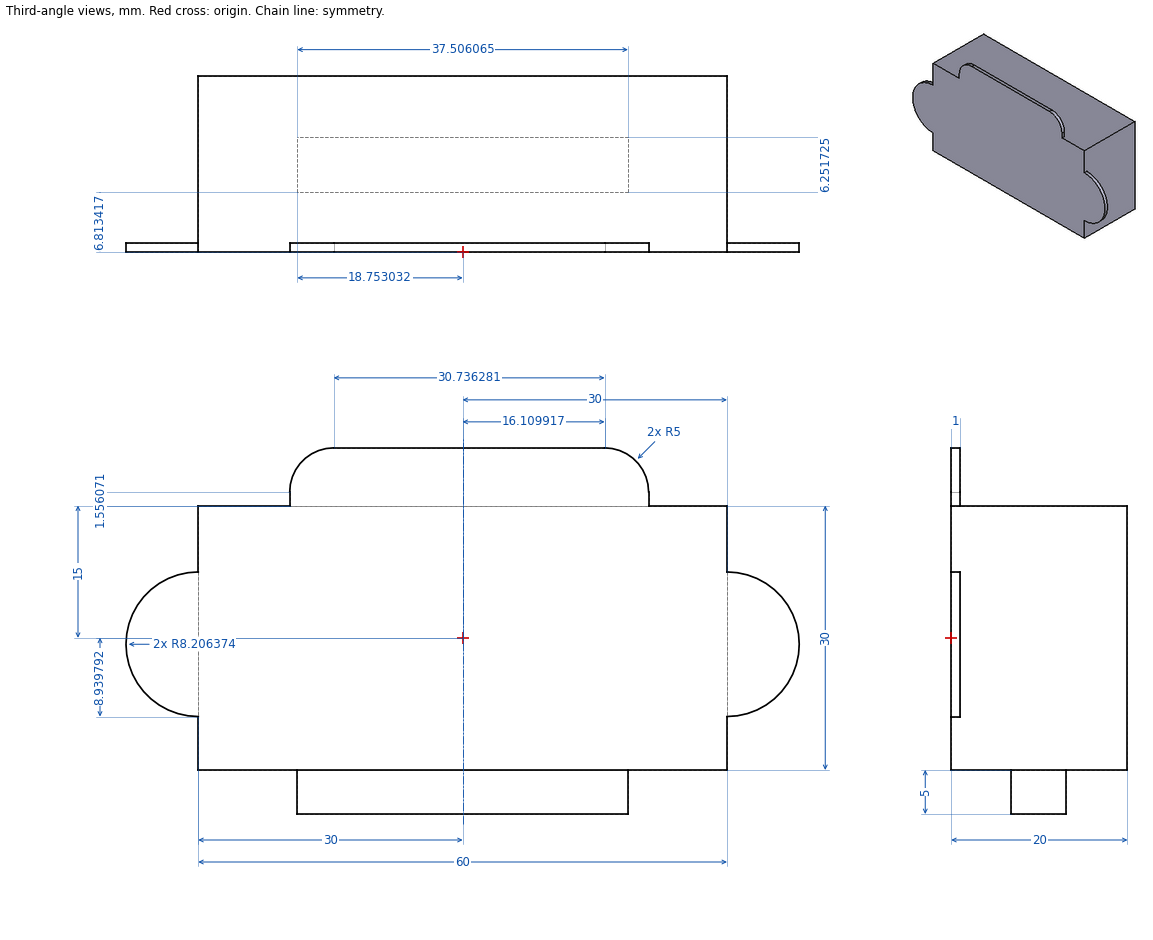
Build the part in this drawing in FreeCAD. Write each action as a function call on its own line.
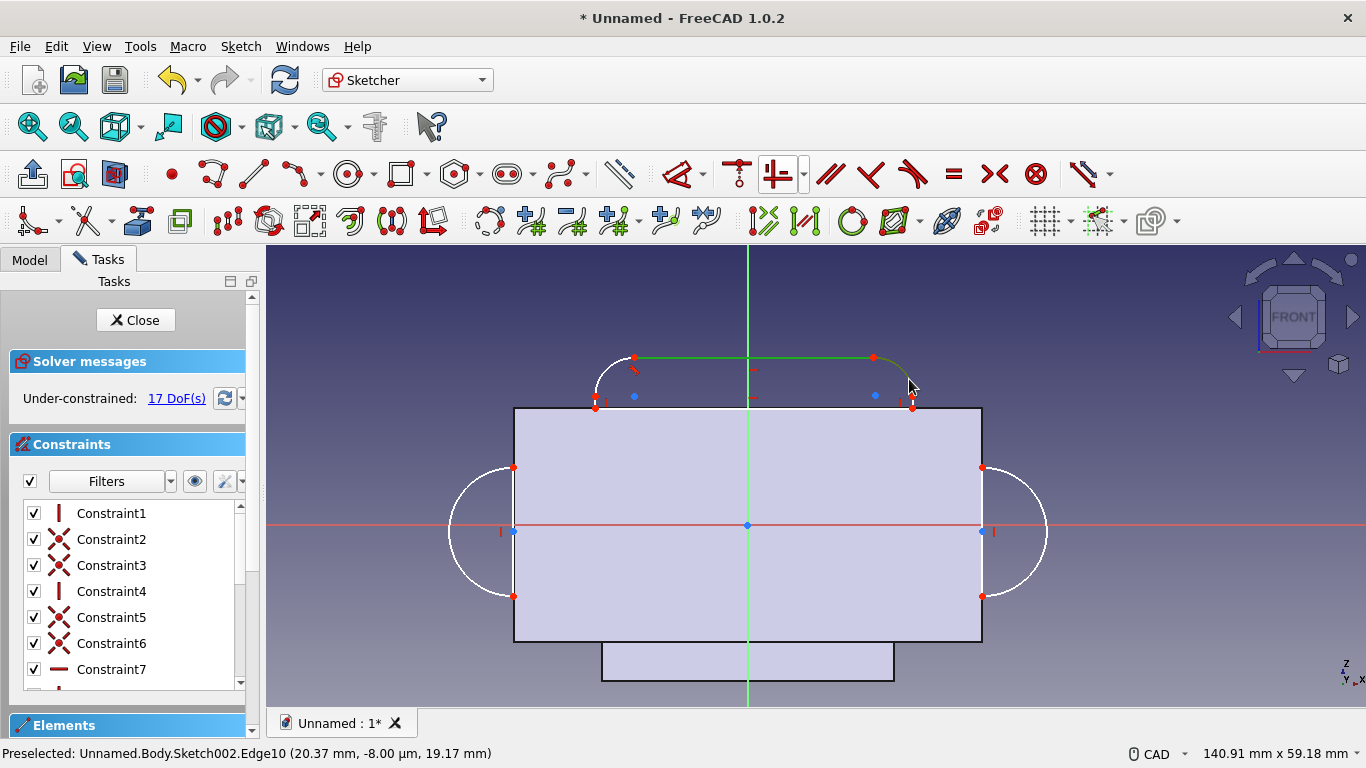
key(t)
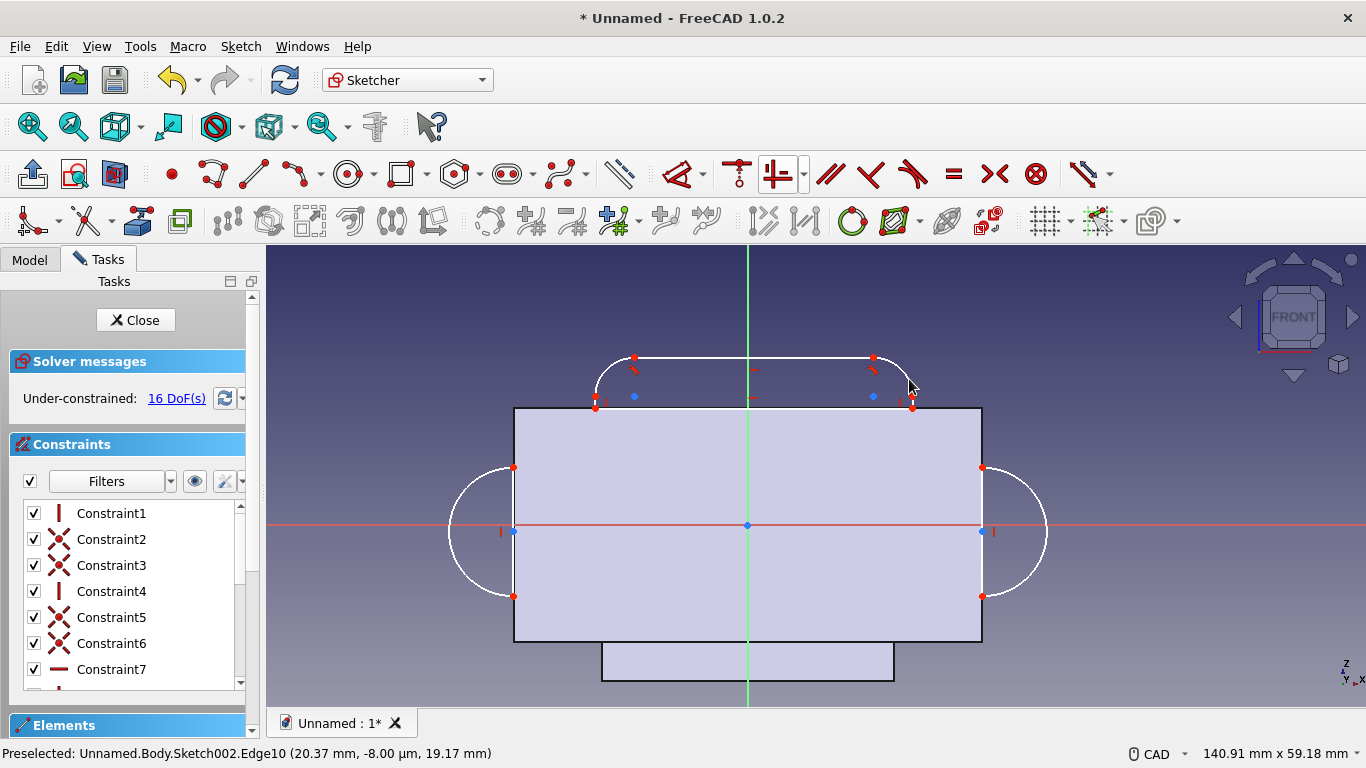
scroll(595, 403, up, 5)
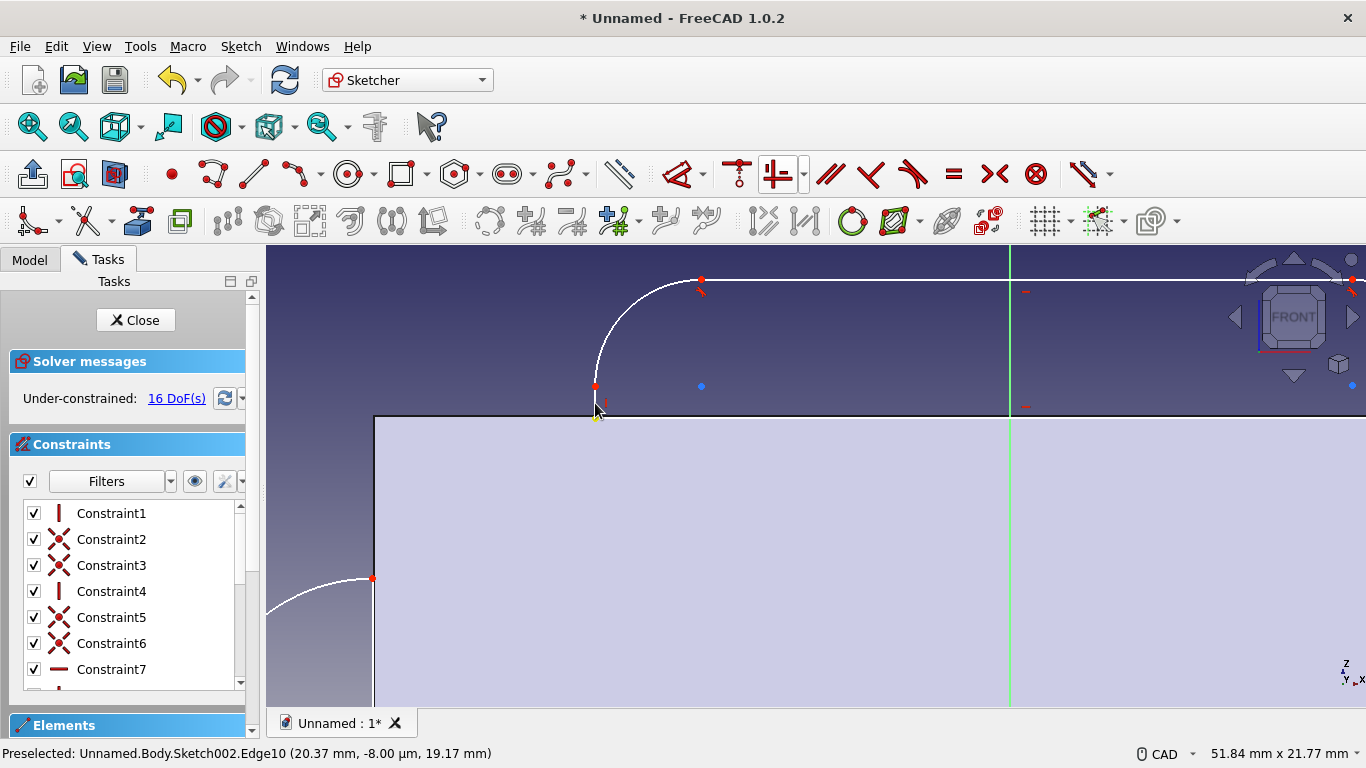
click(595, 402)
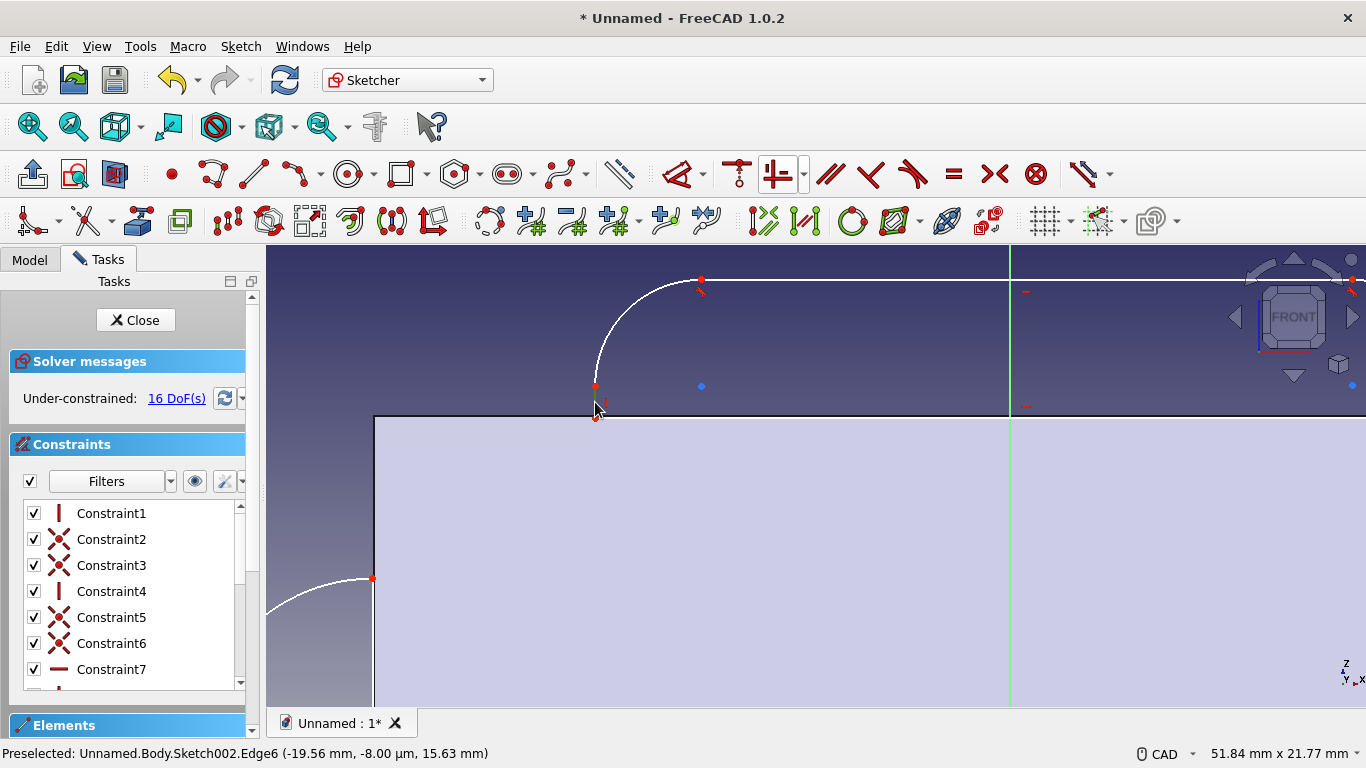
click(653, 291)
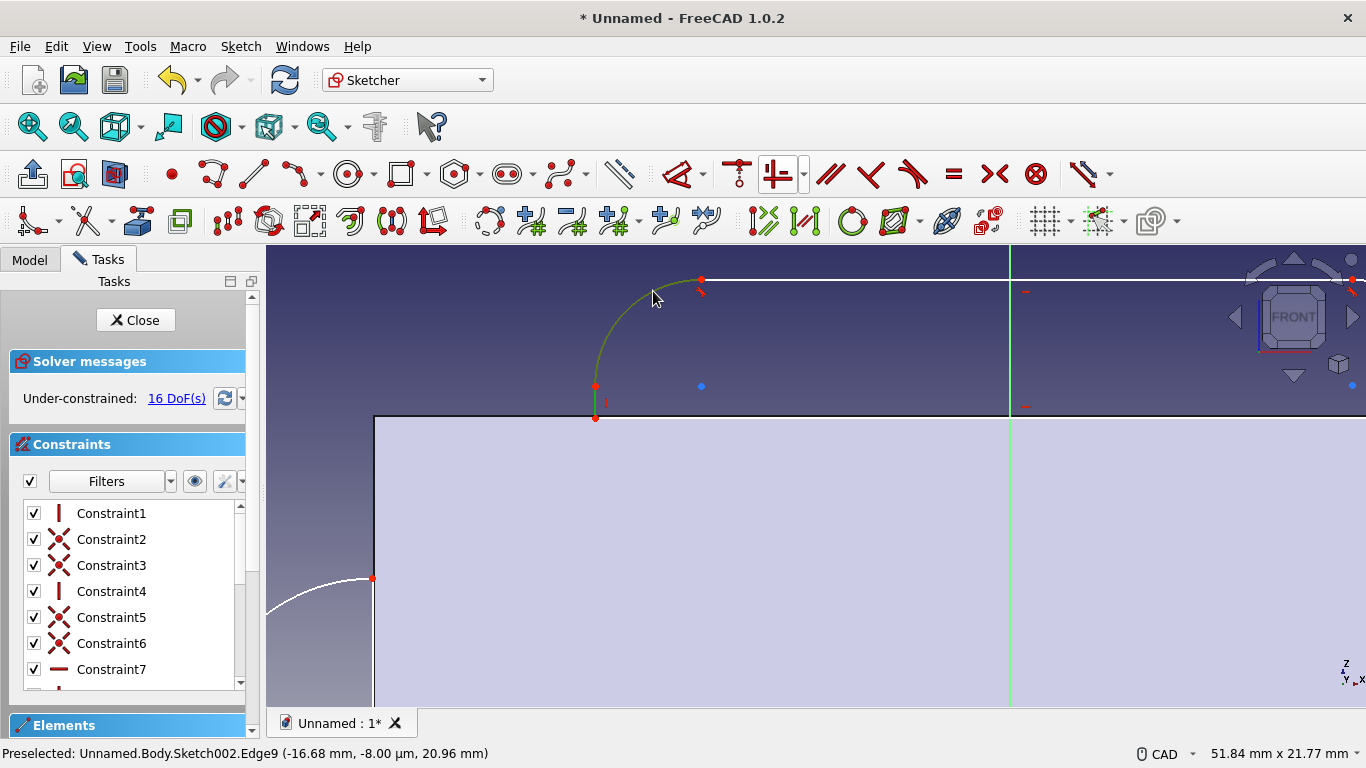
click(913, 174)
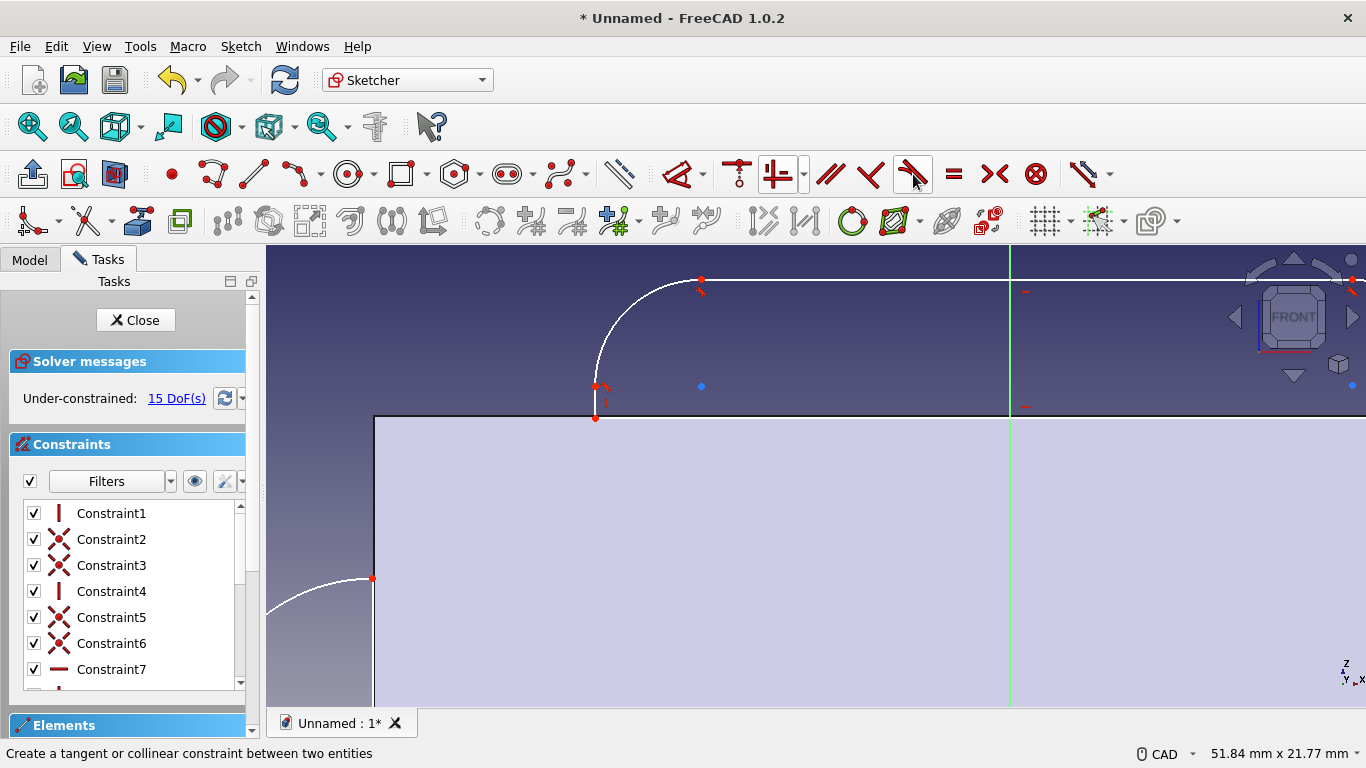
scroll(595, 403, down, 5)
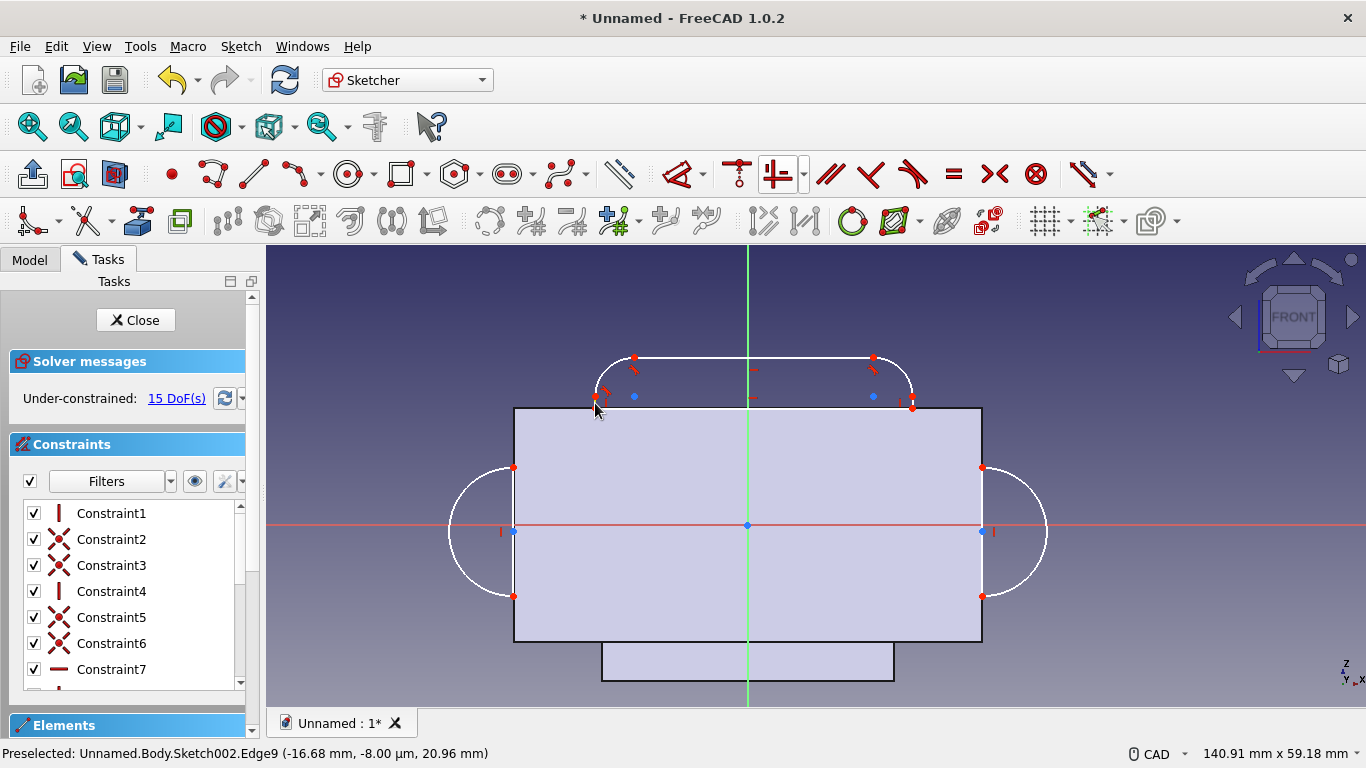
scroll(913, 405, up, 7)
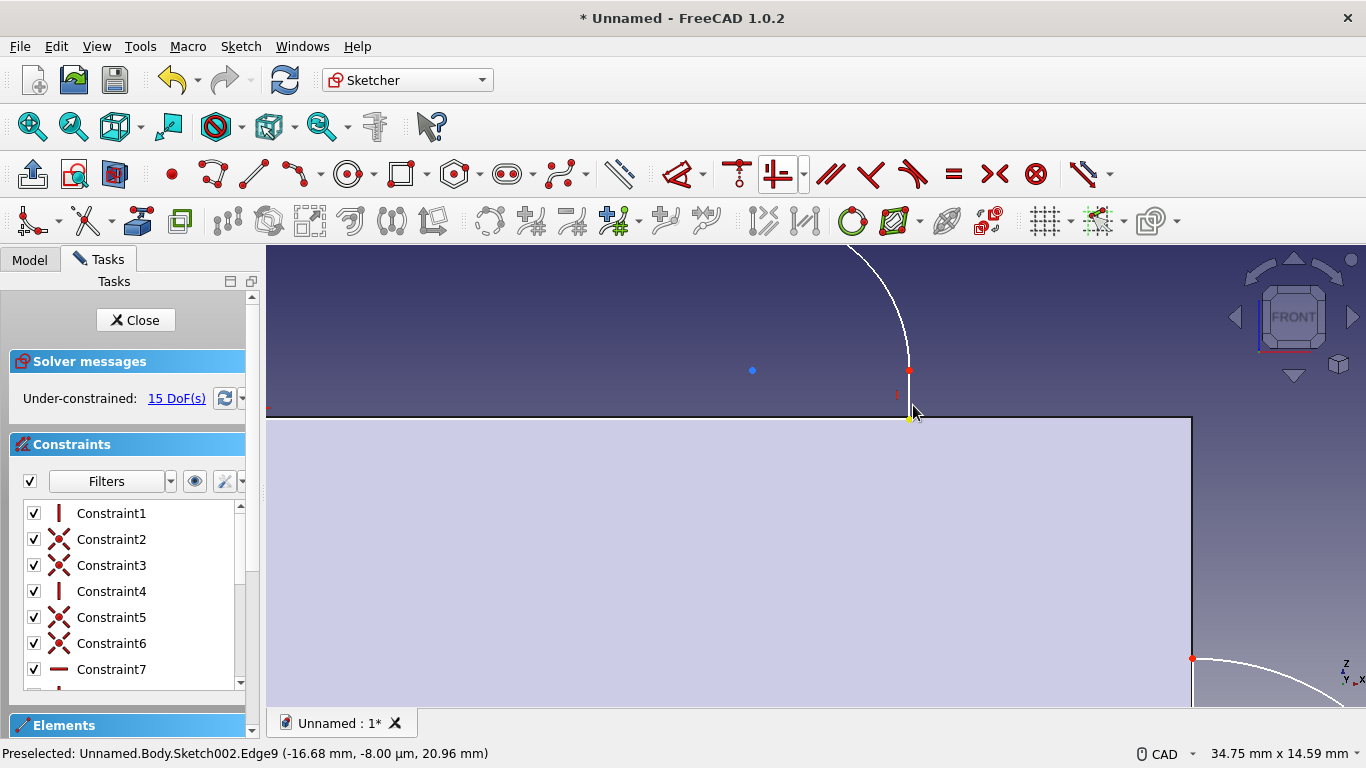
click(909, 405)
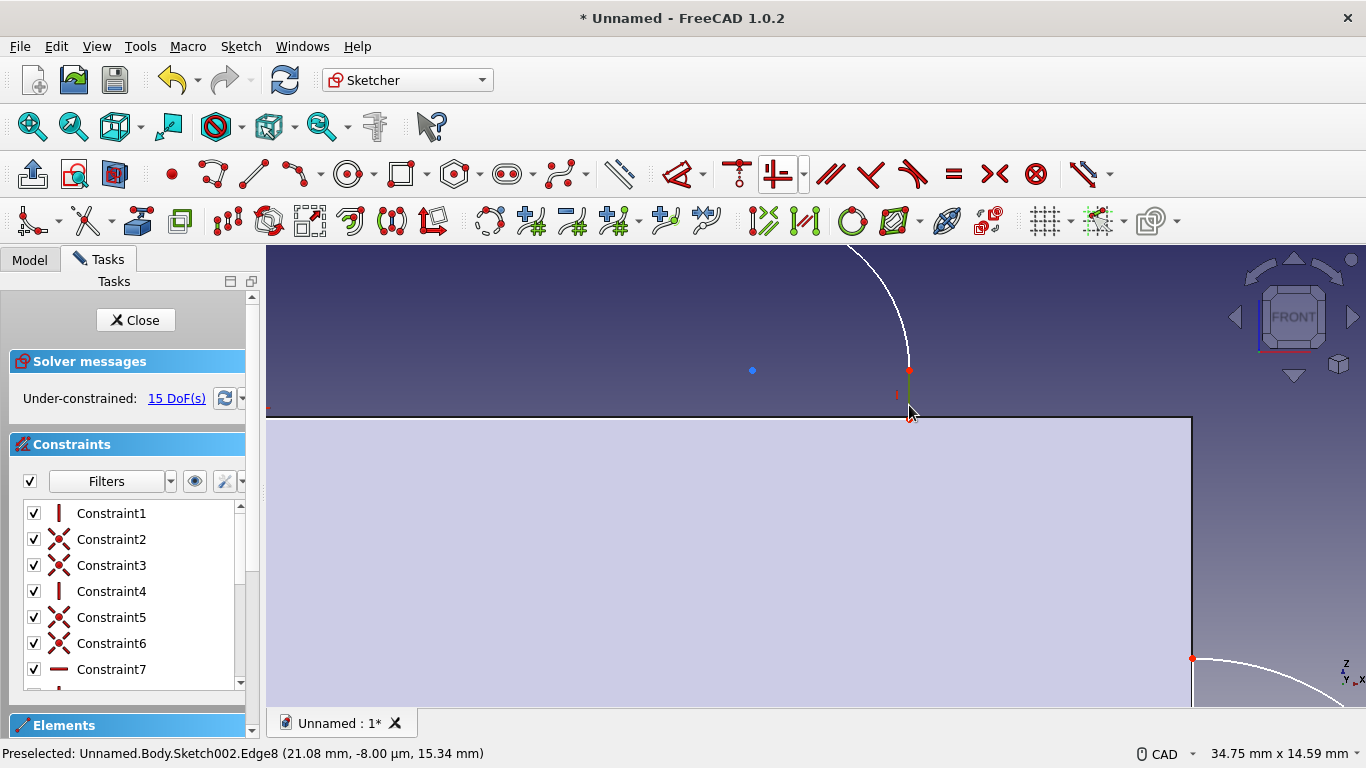
scroll(913, 405, down, 7)